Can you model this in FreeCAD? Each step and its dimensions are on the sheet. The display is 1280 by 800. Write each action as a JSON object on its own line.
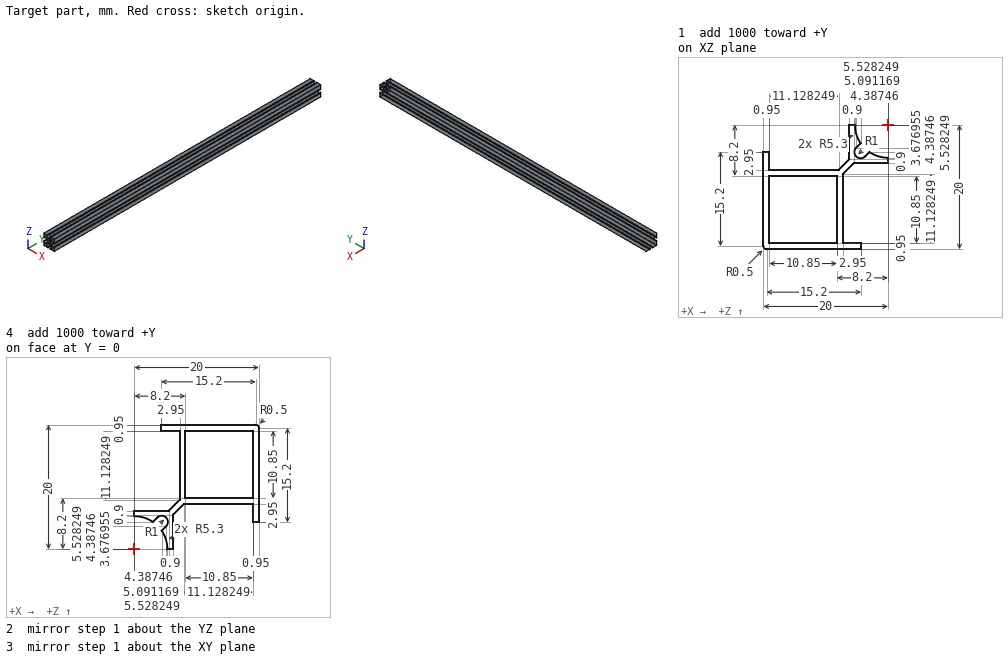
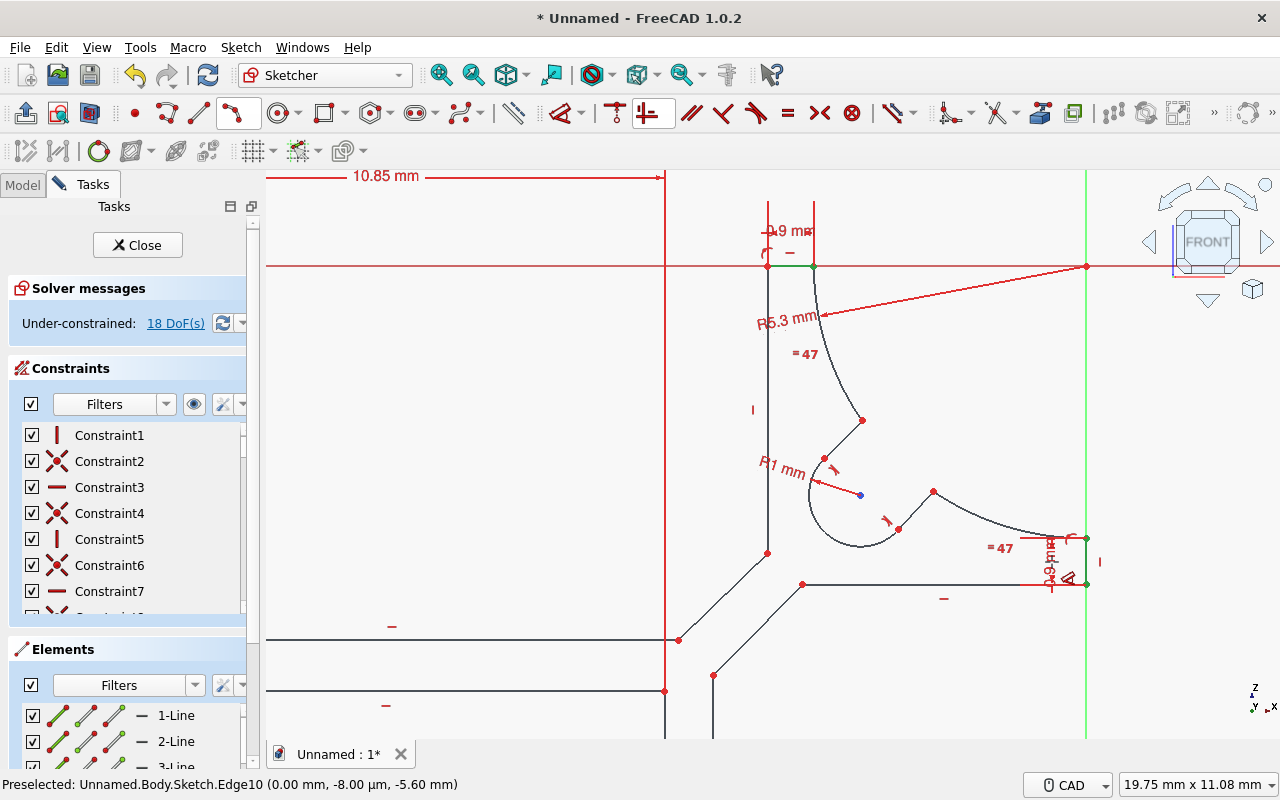
{"action": "scroll", "coordinate": [781, 265], "scroll_direction": "down", "scroll_amount": 5}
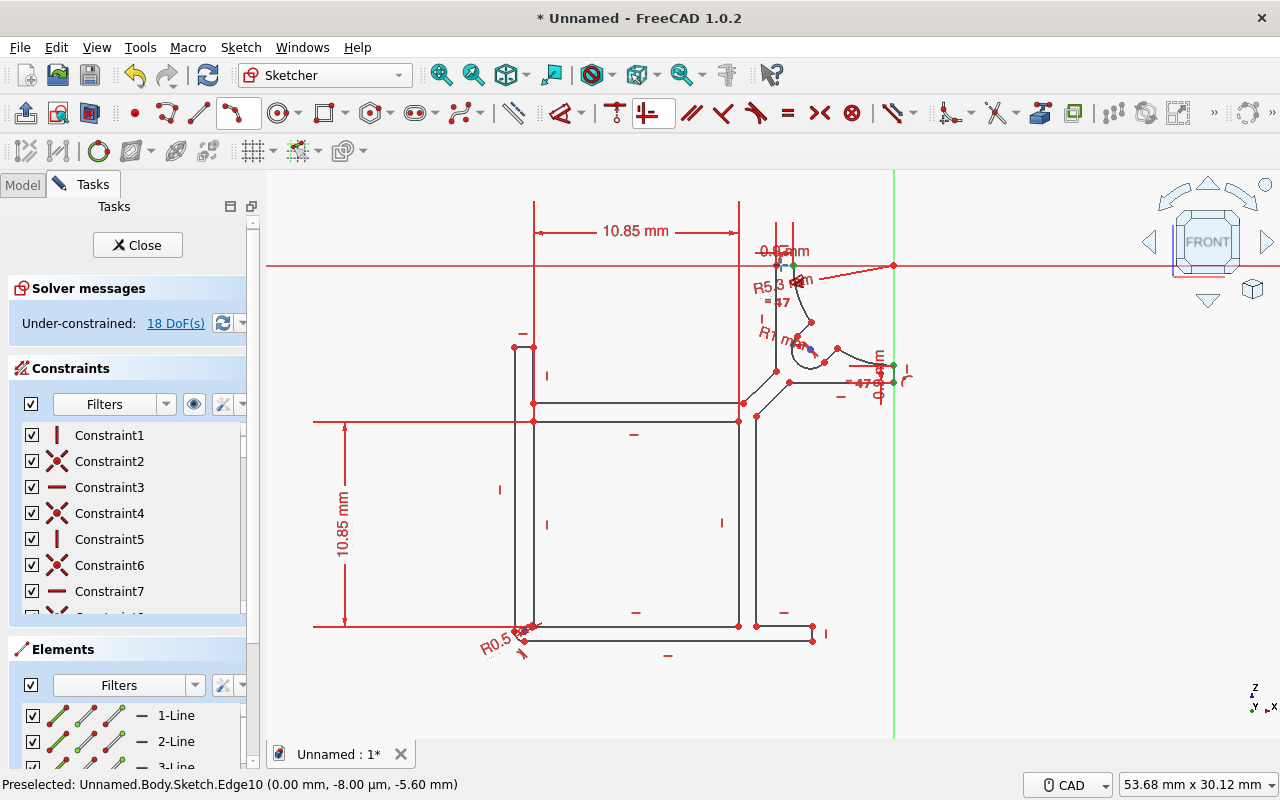
{"action": "scroll", "coordinate": [515, 632], "scroll_direction": "up", "scroll_amount": 2}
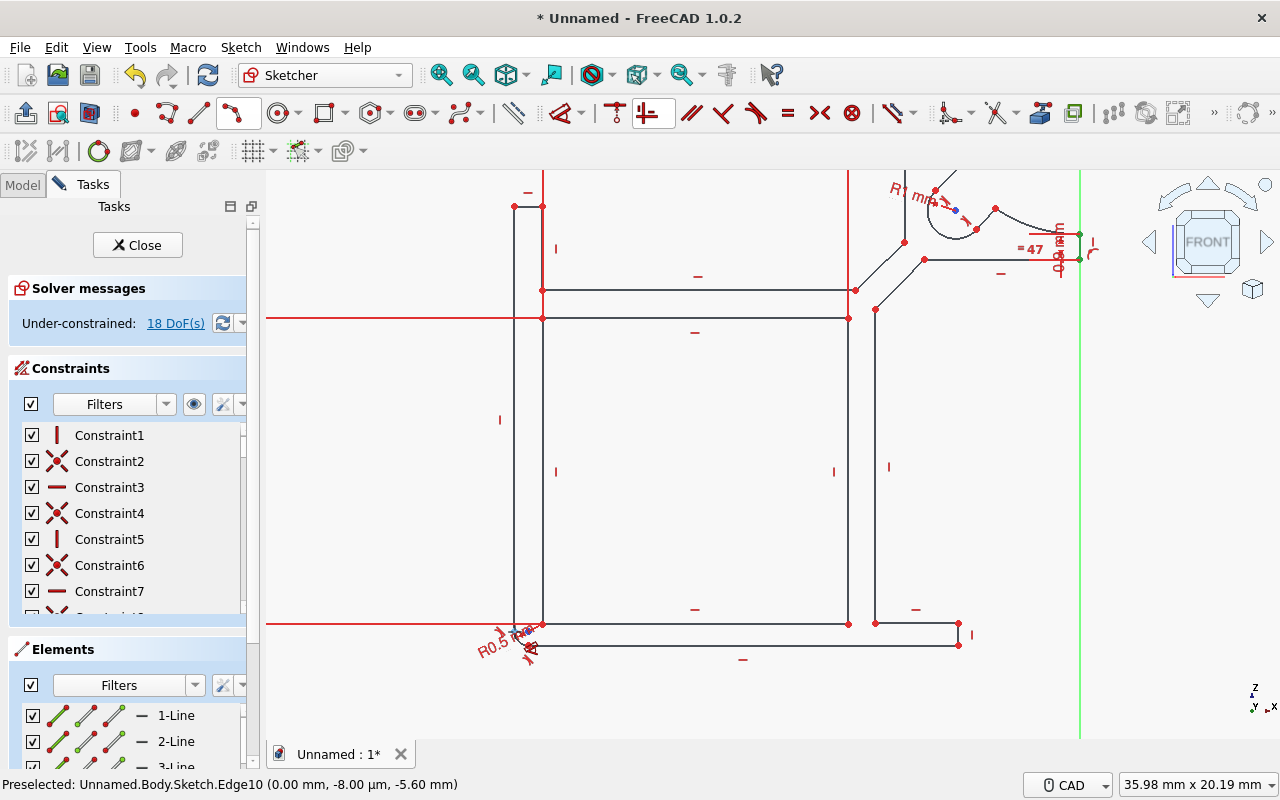
{"action": "left_click", "coordinate": [514, 631]}
{"action": "left_click", "coordinate": [797, 665]}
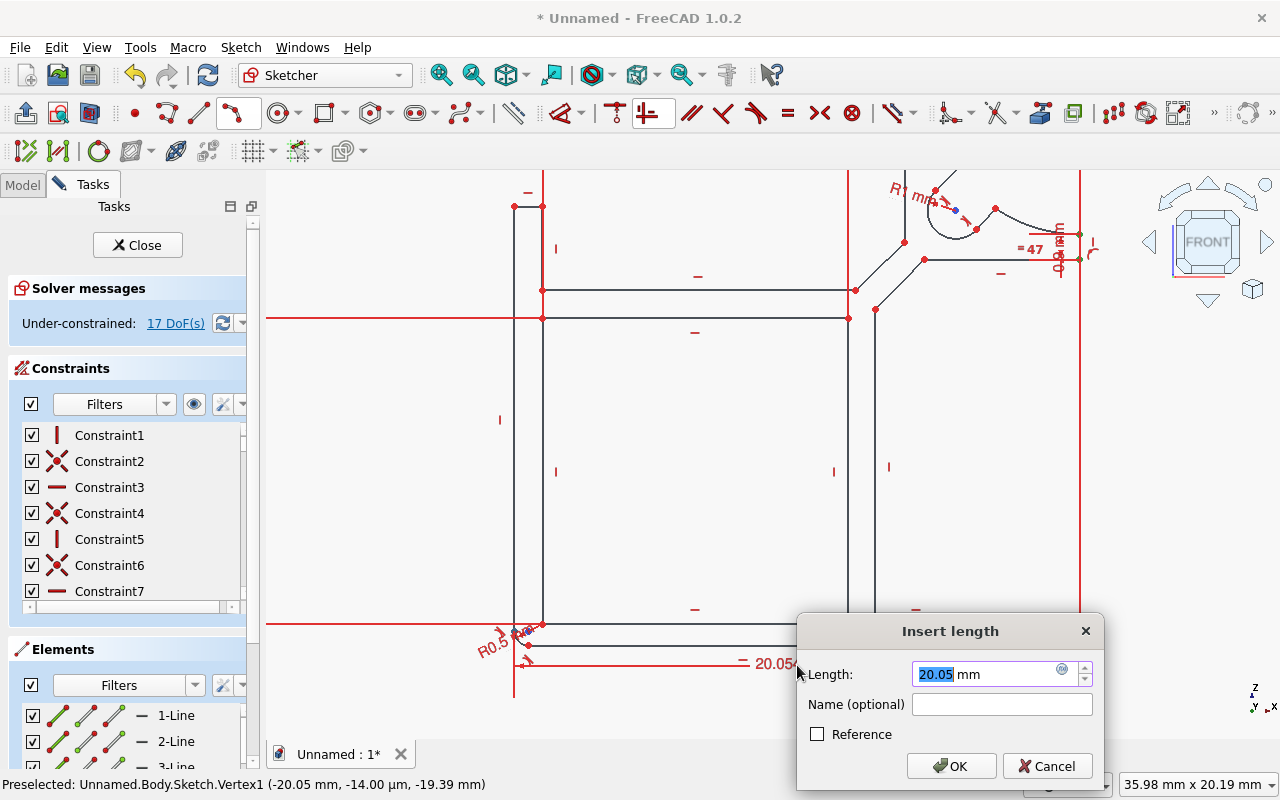
{"action": "type", "text": "20"}
{"action": "key", "text": "Return"}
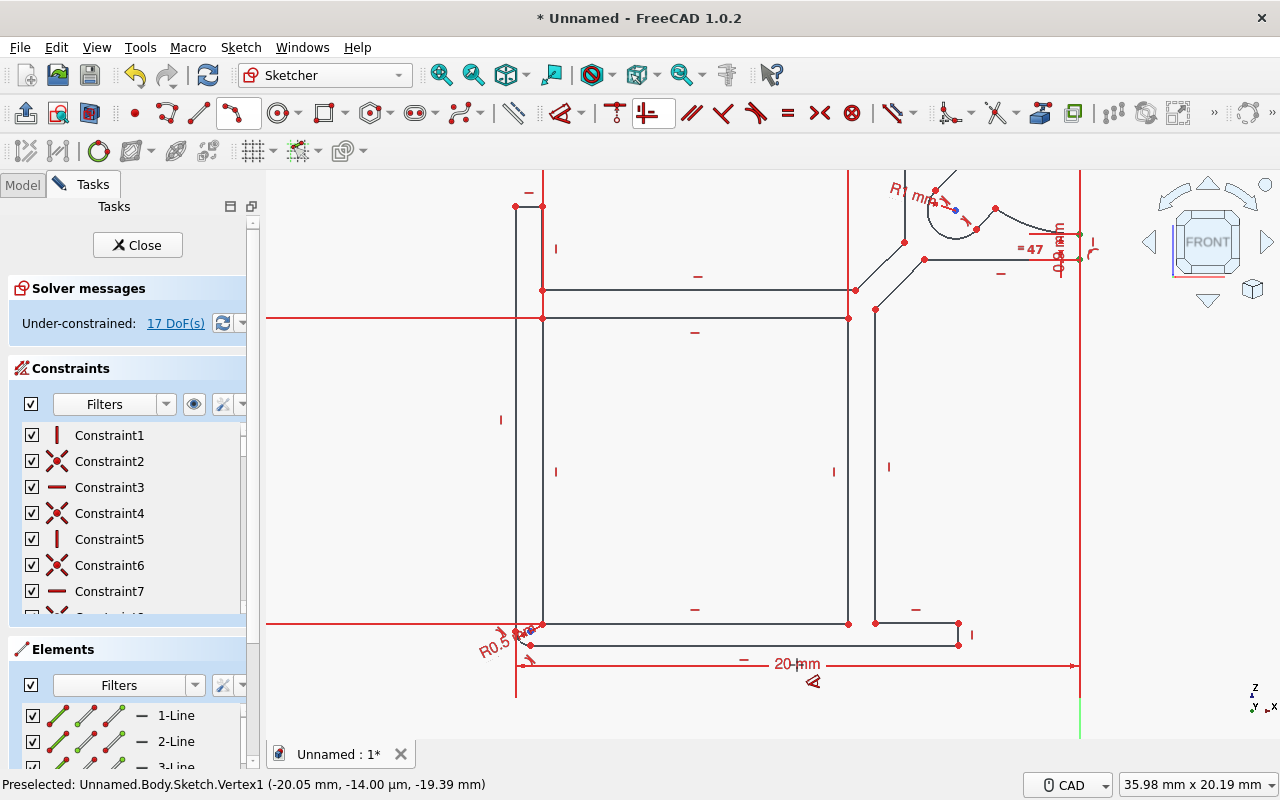
{"action": "left_click", "coordinate": [958, 646]}
{"action": "left_click", "coordinate": [1114, 422]}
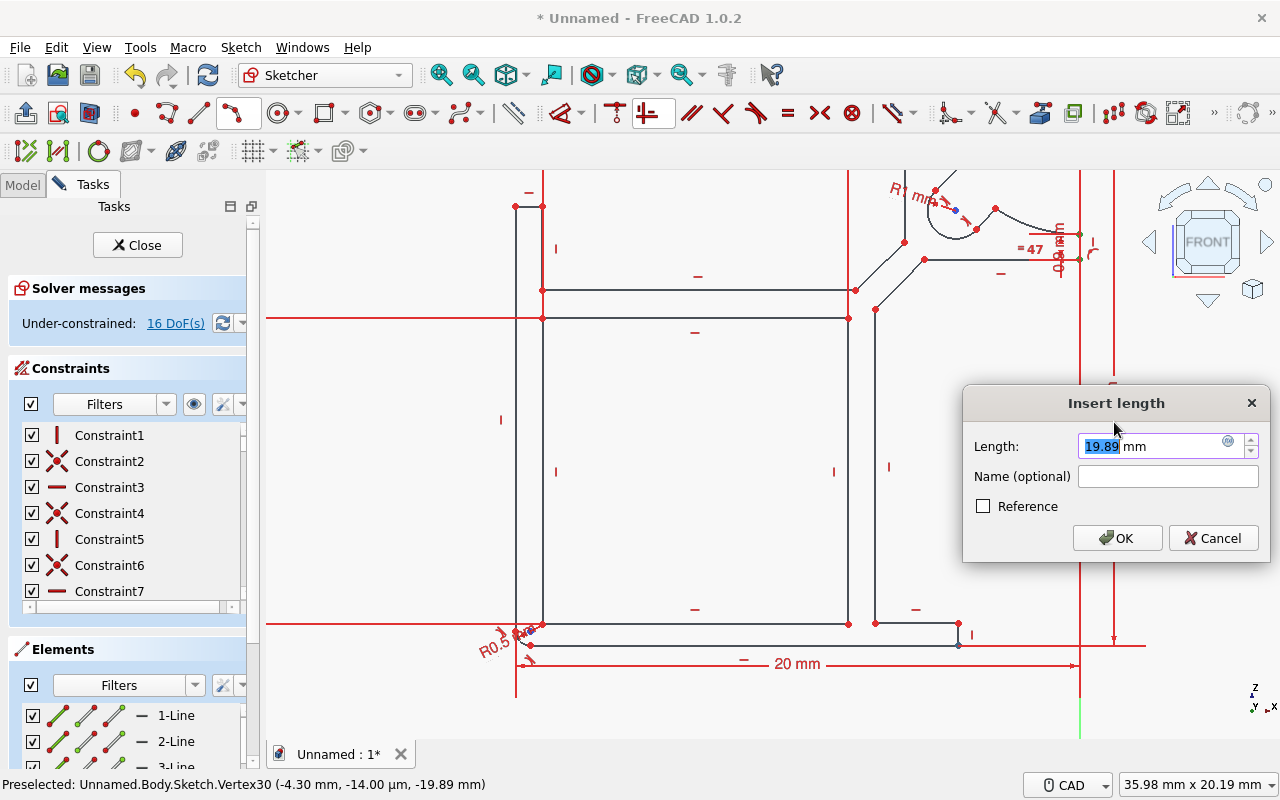
{"action": "type", "text": "20"}
{"action": "key", "text": "Return"}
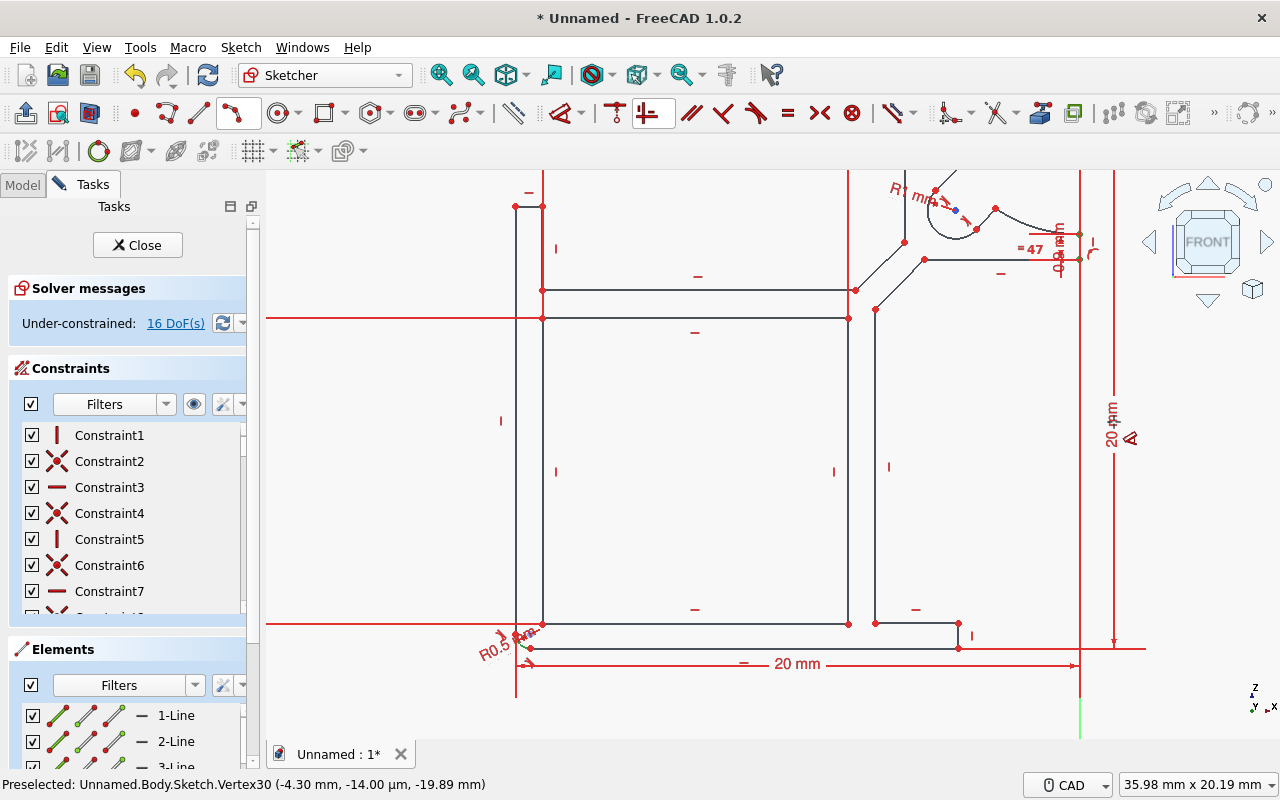
{"action": "left_click", "coordinate": [516, 506]}
{"action": "left_click", "coordinate": [482, 421]}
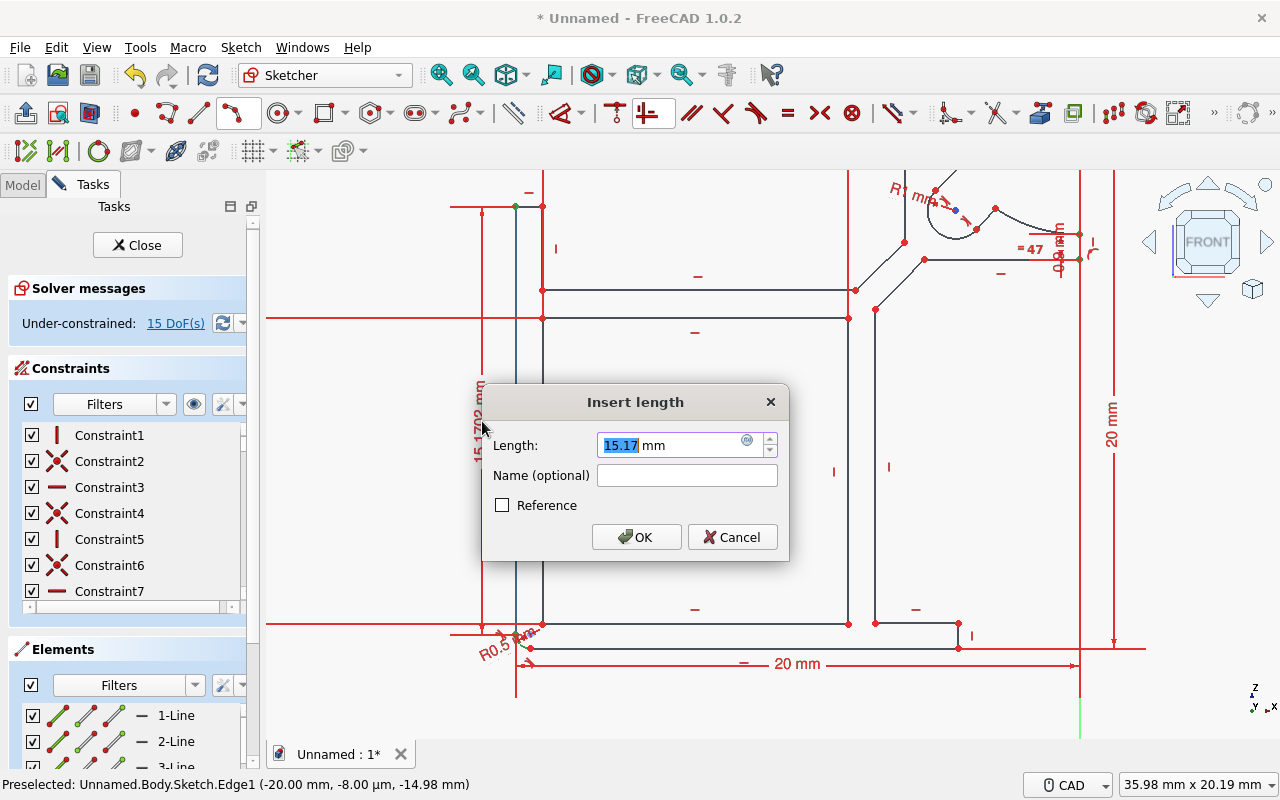
{"action": "type", "text": "15.2"}
{"action": "key", "text": "Return"}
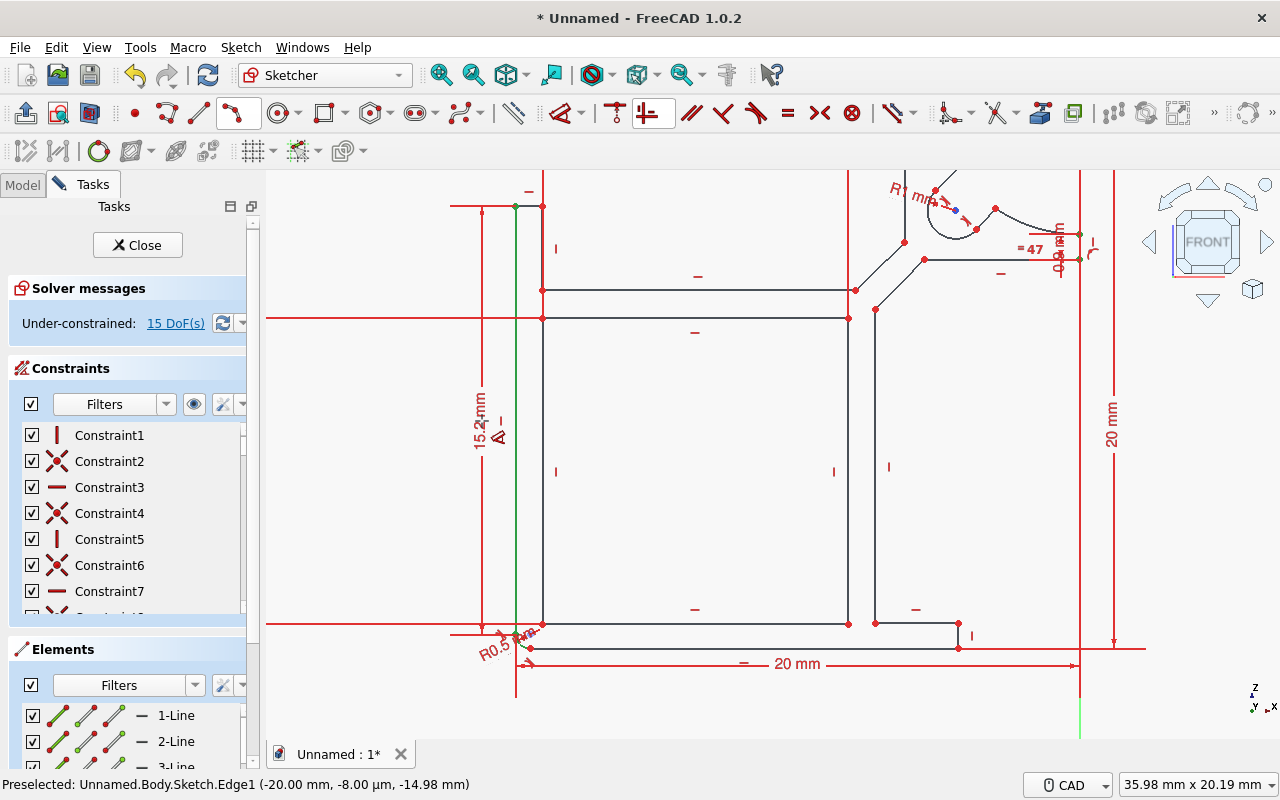
{"action": "scroll", "coordinate": [526, 206], "scroll_direction": "up", "scroll_amount": 2}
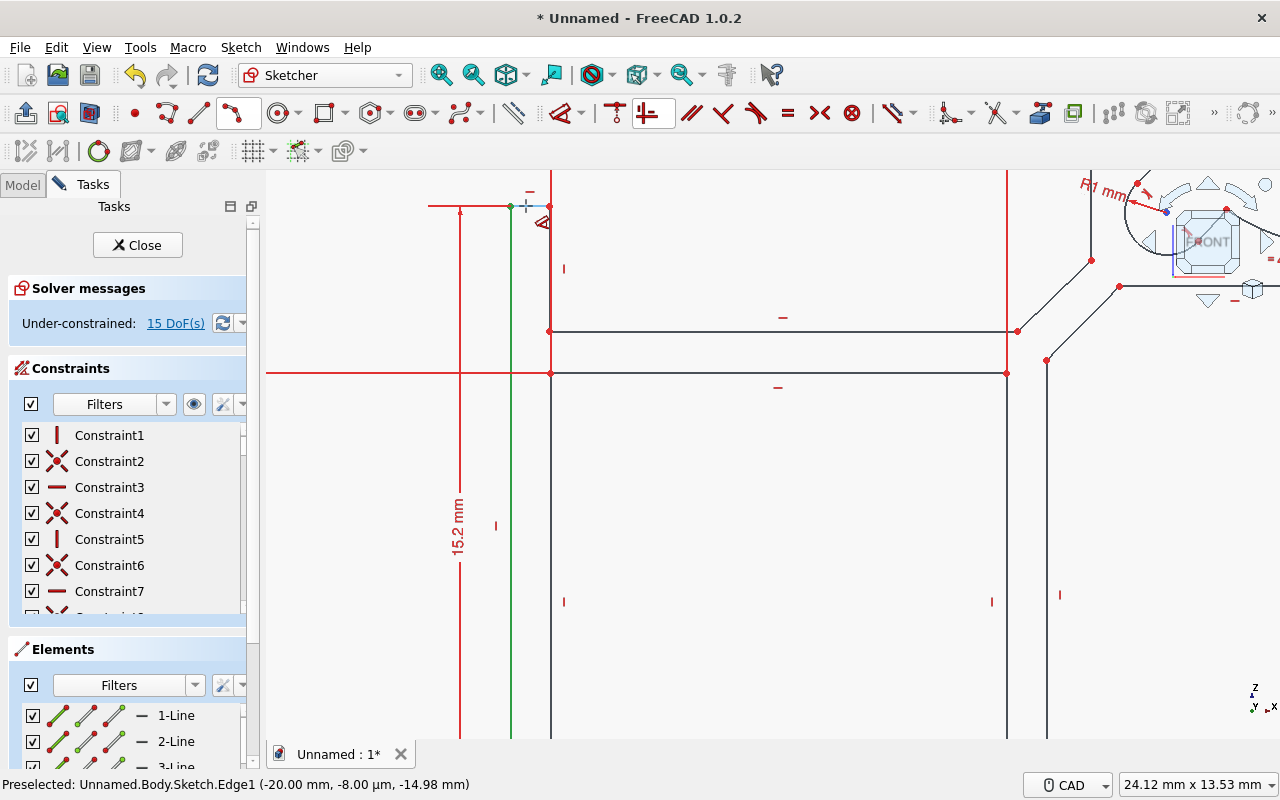
{"action": "left_click", "coordinate": [526, 206]}
{"action": "left_click", "coordinate": [530, 240]}